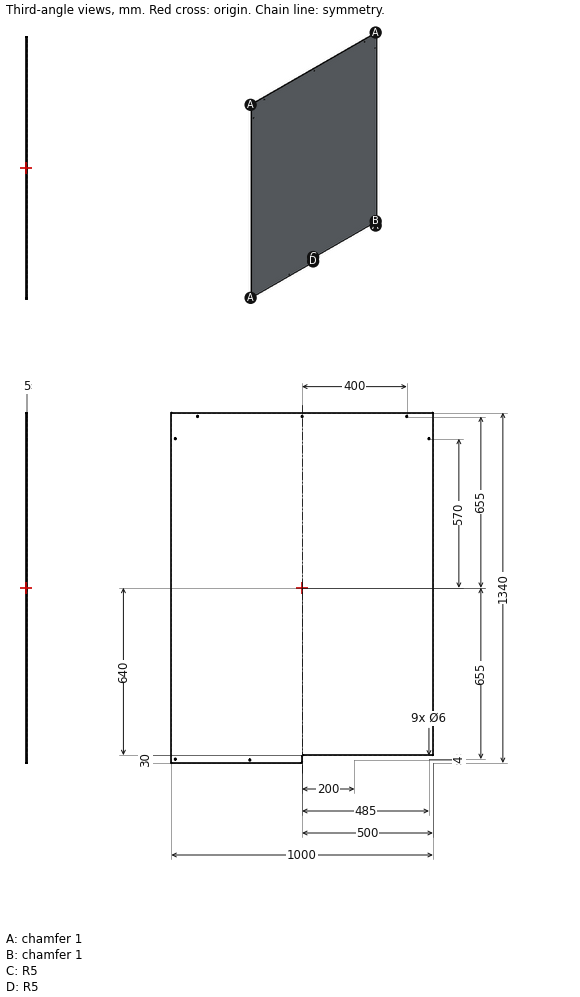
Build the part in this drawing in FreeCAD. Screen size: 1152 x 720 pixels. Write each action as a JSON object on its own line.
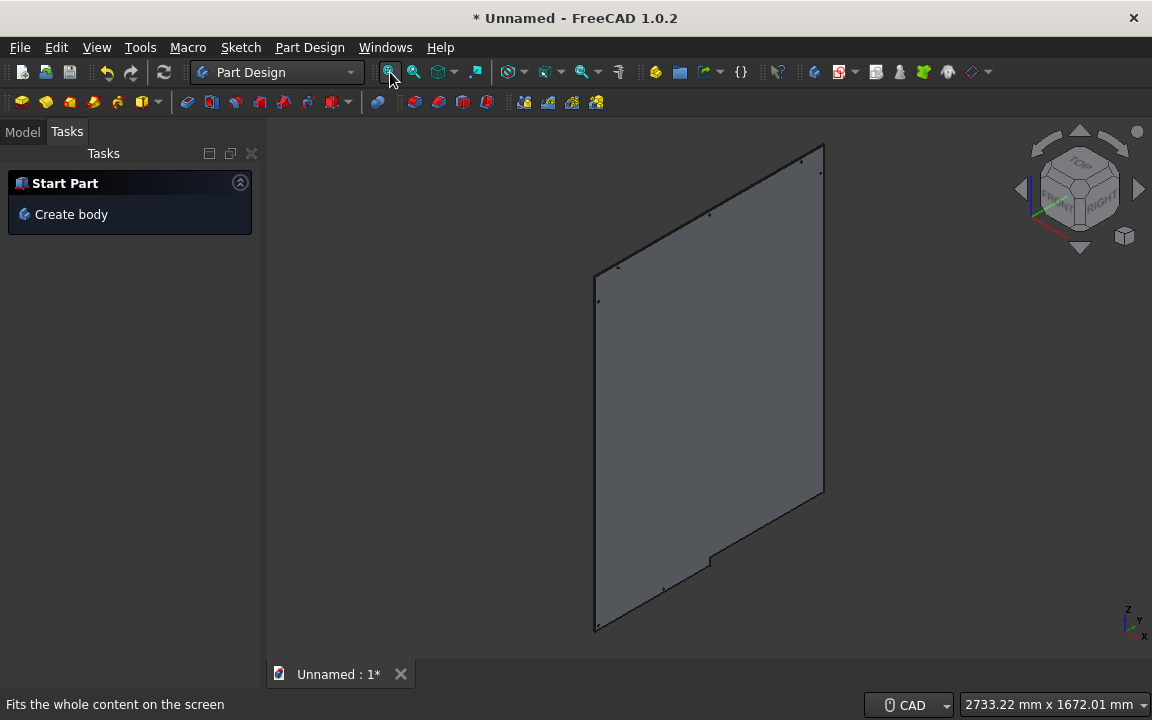
{"action": "scroll", "coordinate": [709, 556], "scroll_direction": "up", "scroll_amount": 15}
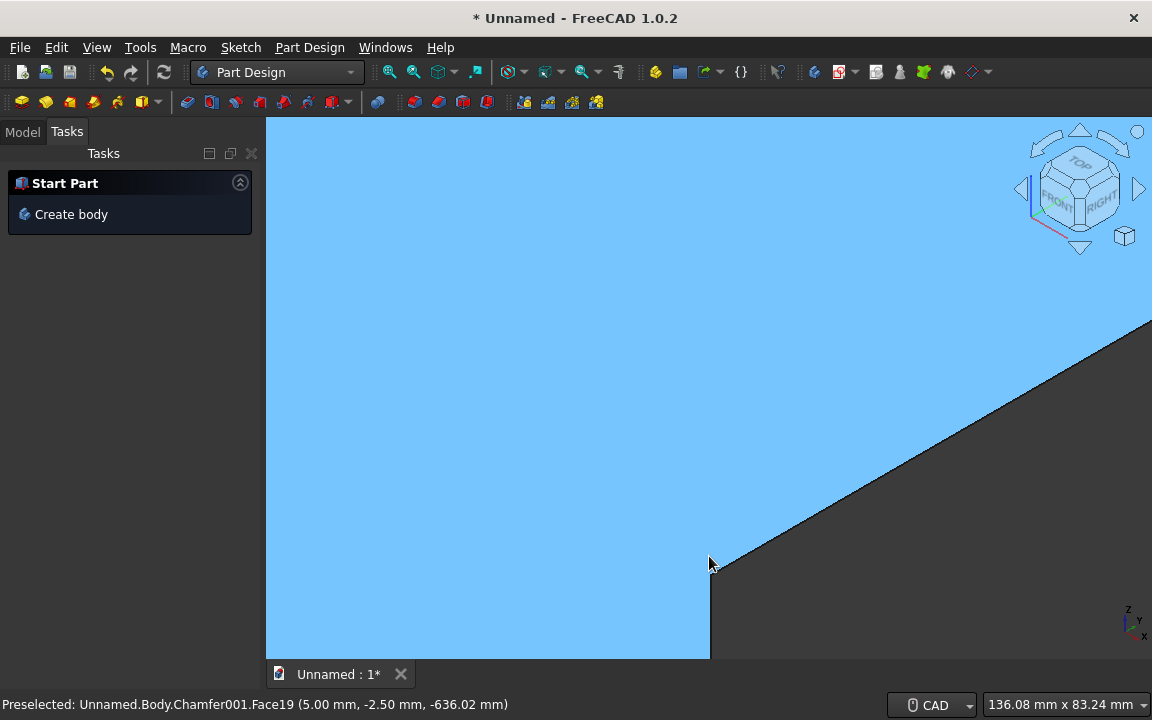
{"action": "left_click", "coordinate": [390, 72]}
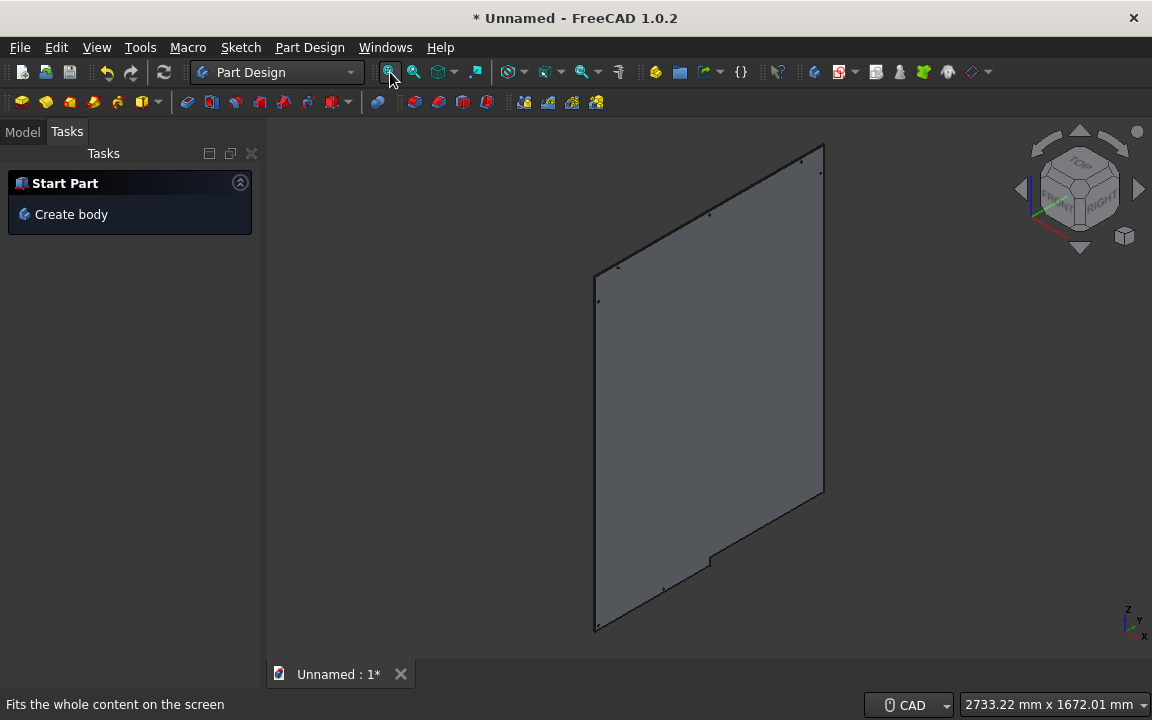
{"action": "key", "text": "2"}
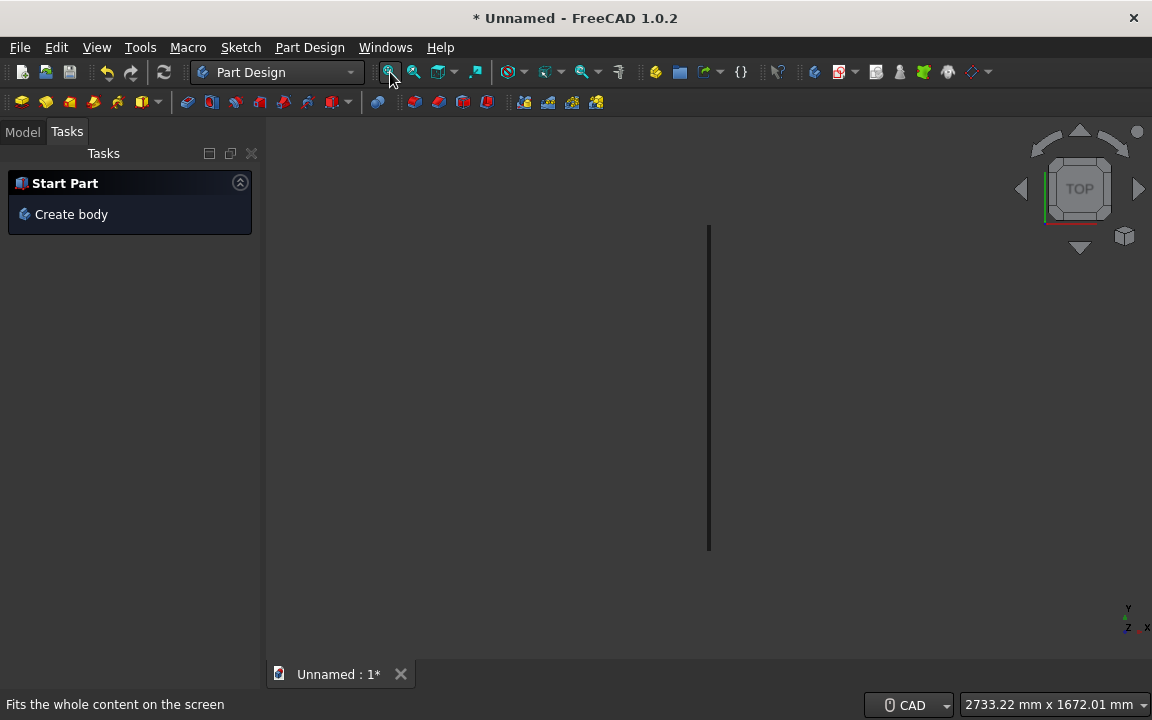
{"action": "scroll", "coordinate": [709, 387], "scroll_direction": "up", "scroll_amount": 15}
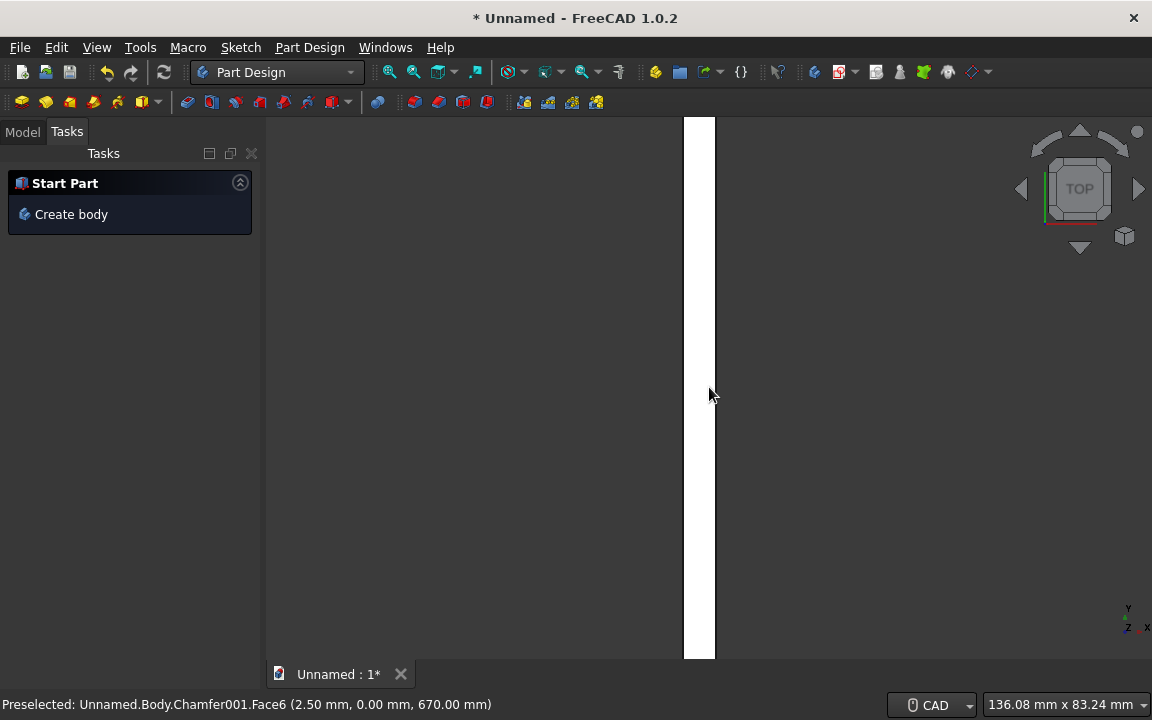
{"action": "left_click", "coordinate": [390, 72]}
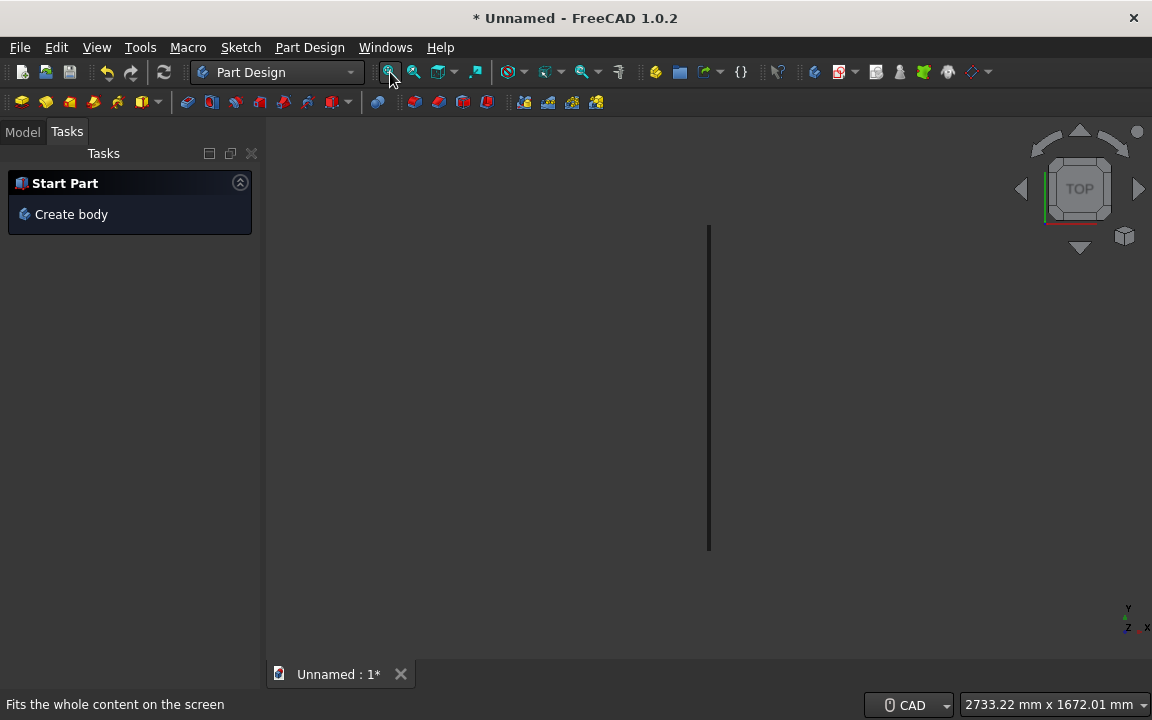
{"action": "key", "text": "1"}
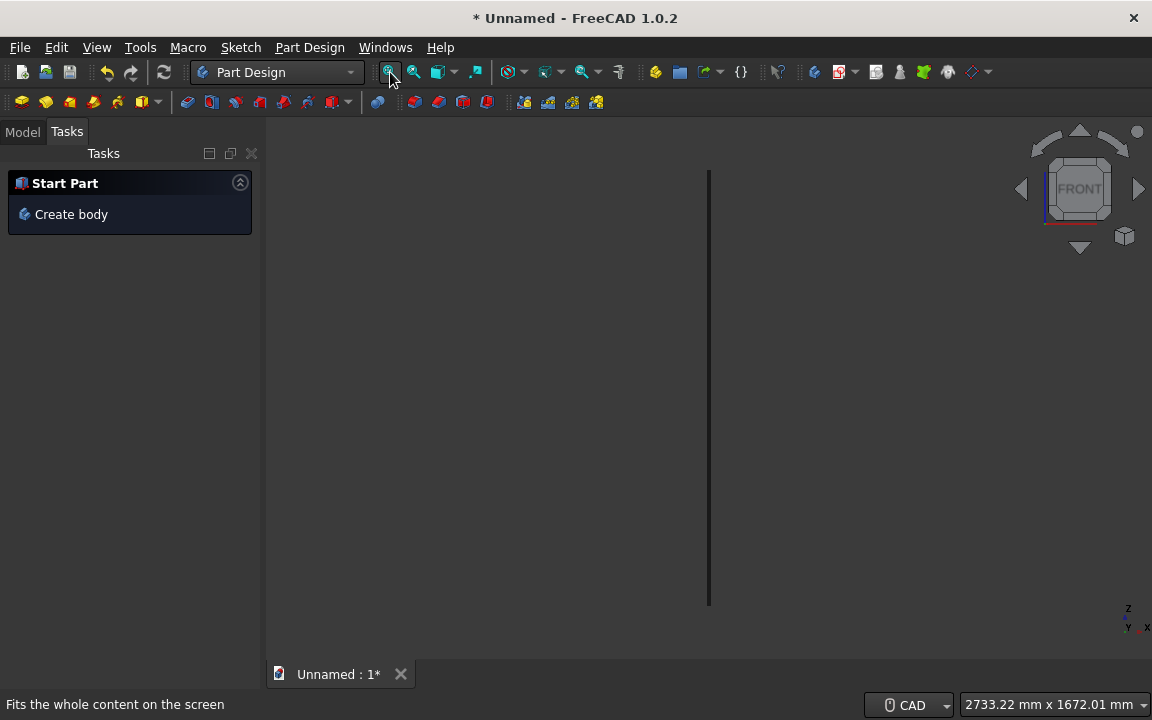
{"action": "scroll", "coordinate": [709, 594], "scroll_direction": "up", "scroll_amount": 15}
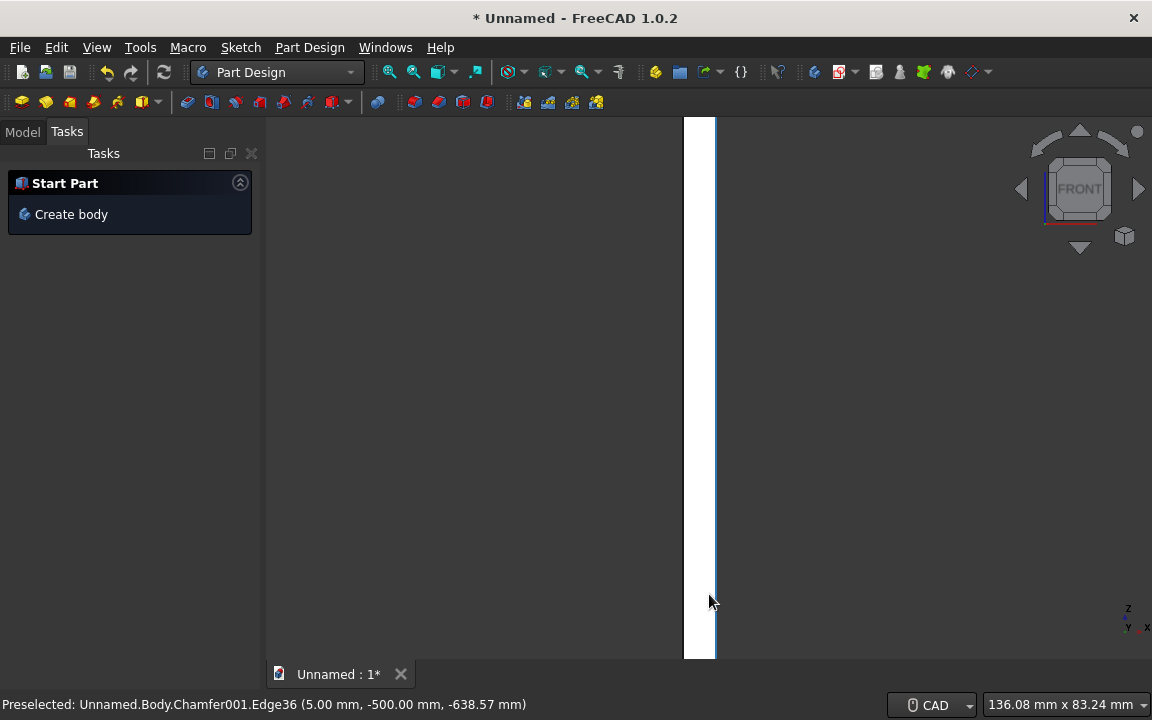
{"action": "left_click", "coordinate": [390, 72]}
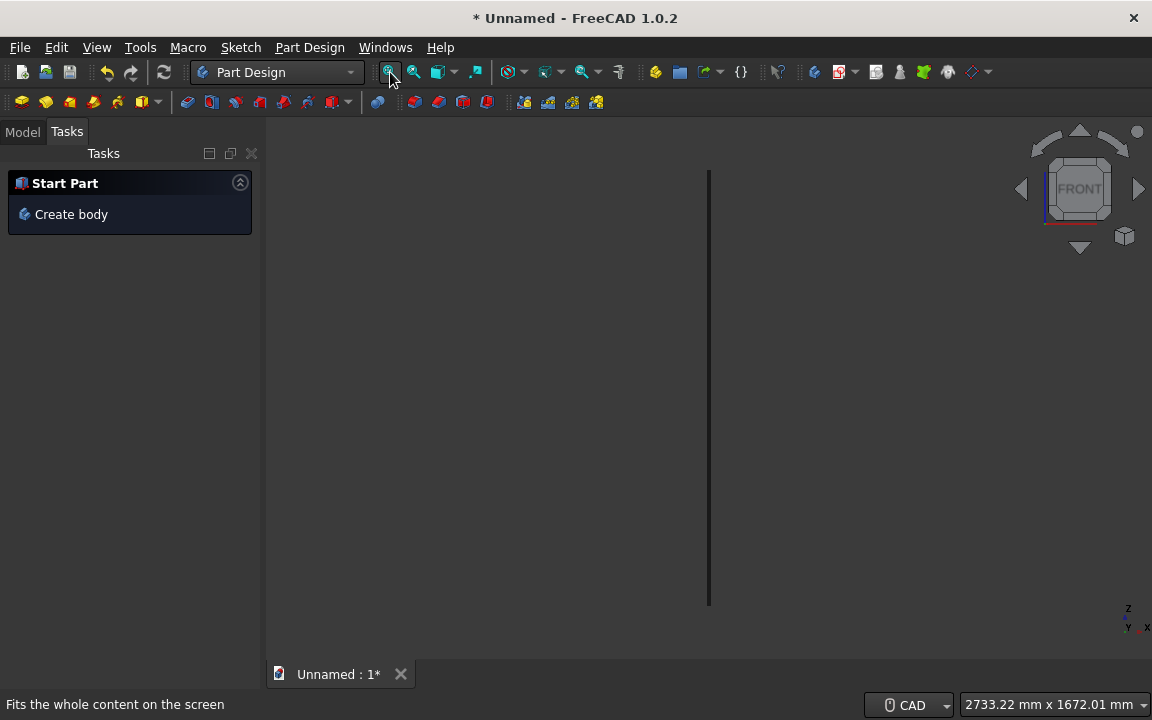
{"action": "key", "text": "3"}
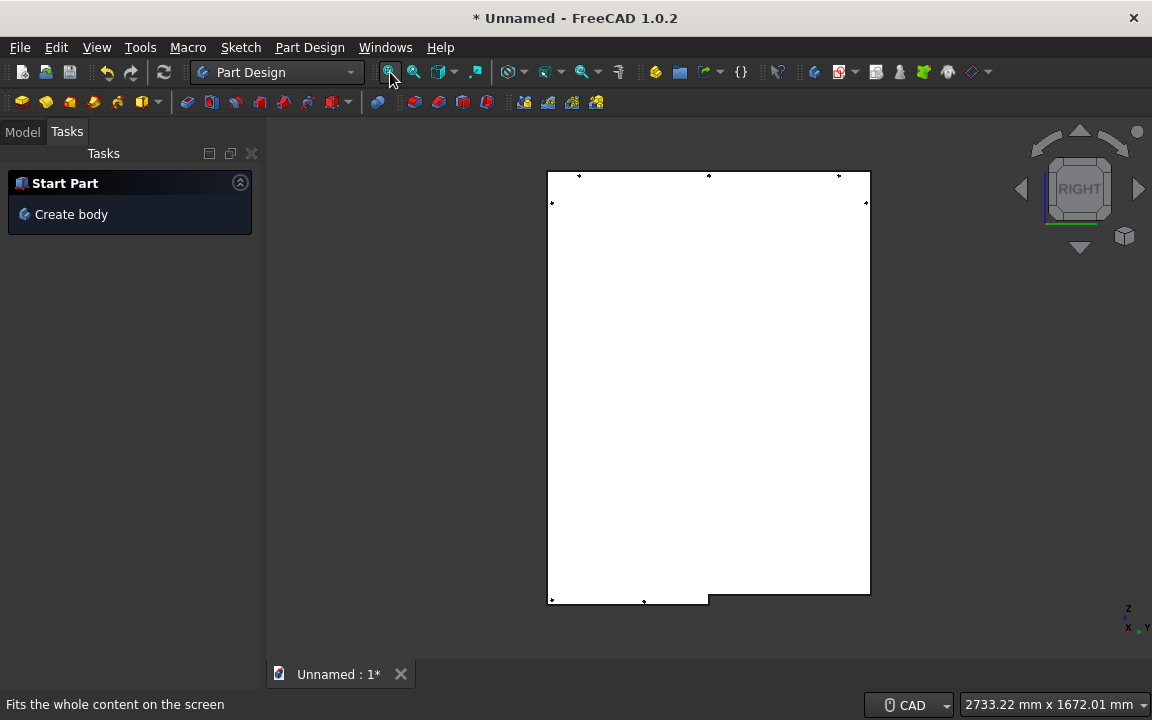
{"action": "scroll", "coordinate": [709, 594], "scroll_direction": "up", "scroll_amount": 15}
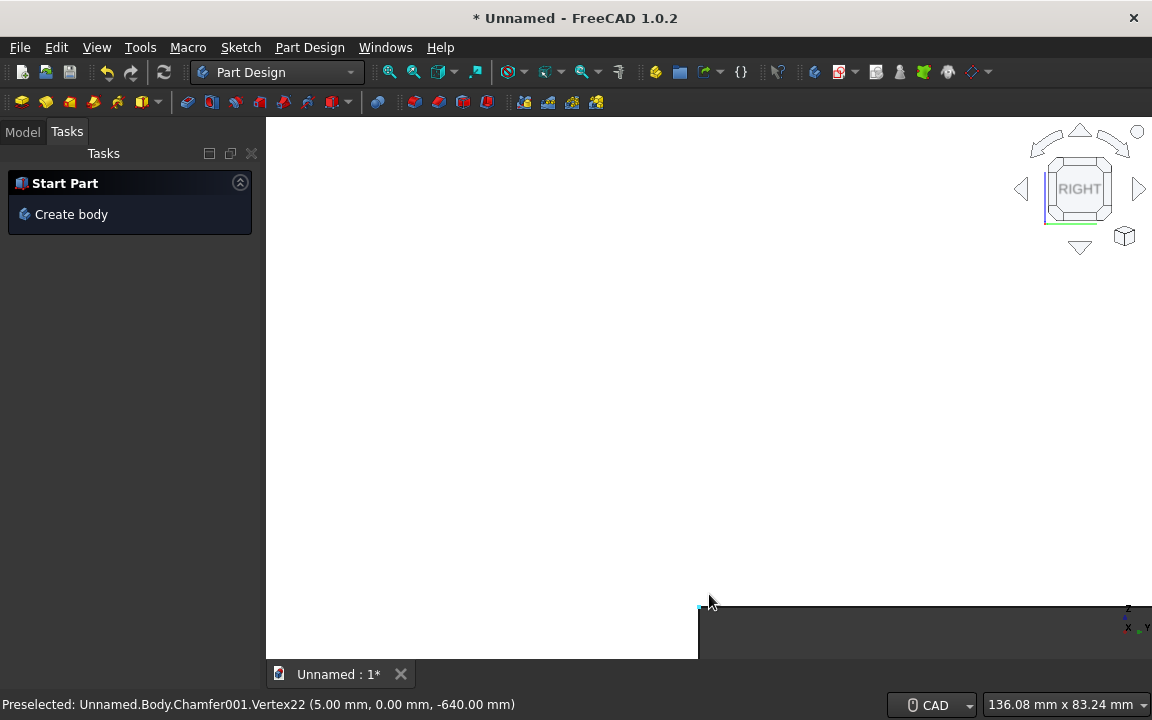
{"action": "left_click", "coordinate": [390, 72]}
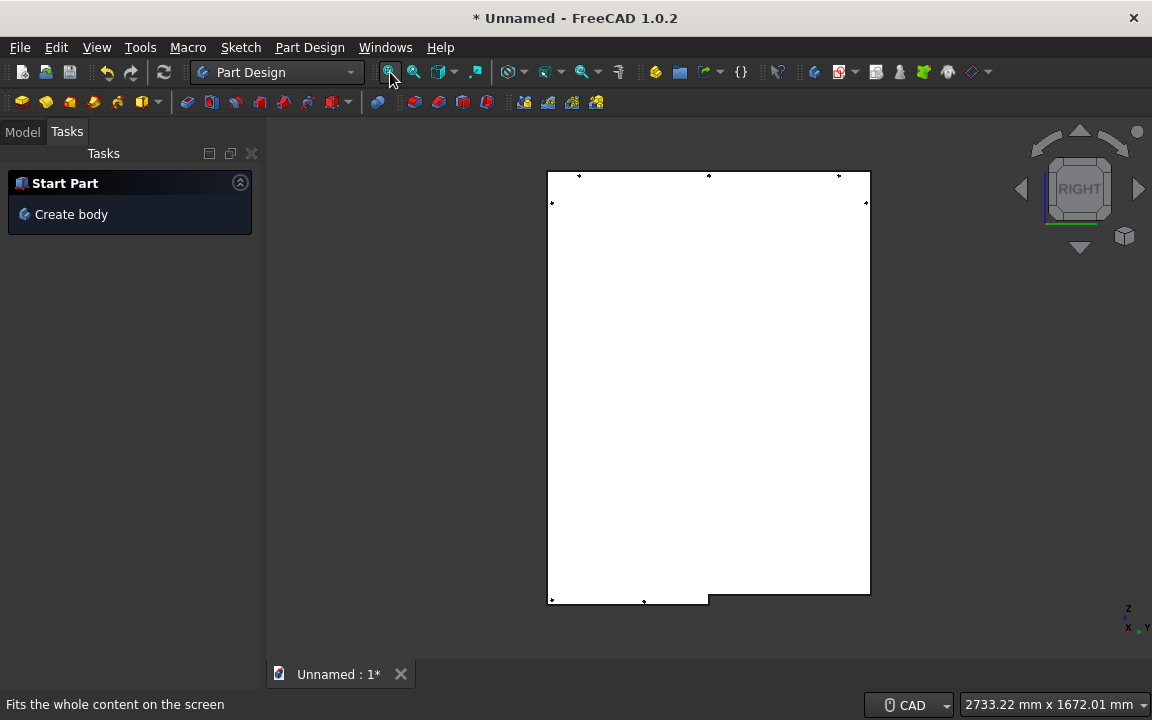
{"action": "key", "text": "5"}